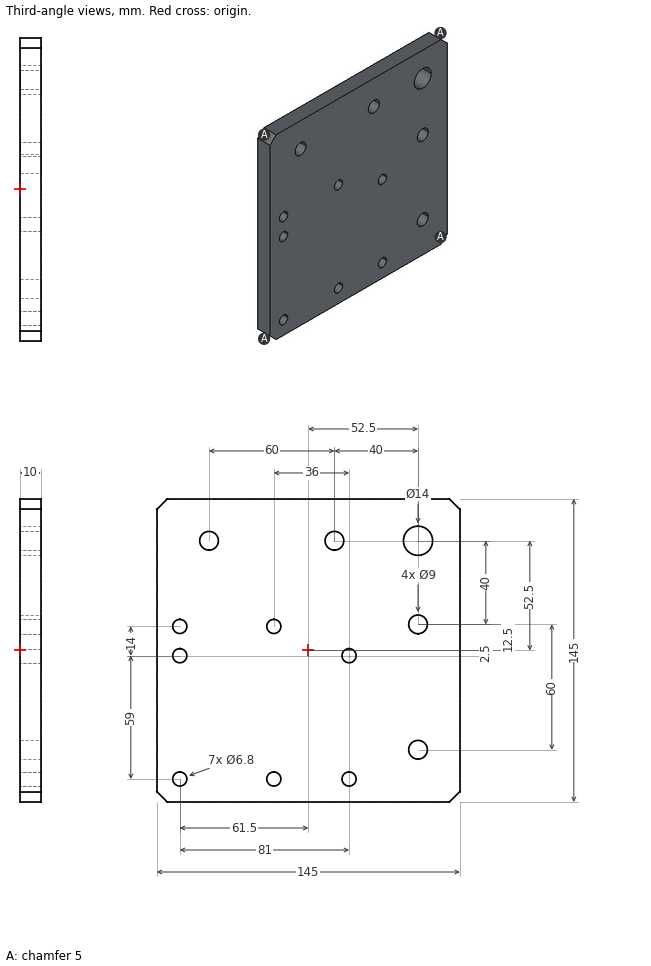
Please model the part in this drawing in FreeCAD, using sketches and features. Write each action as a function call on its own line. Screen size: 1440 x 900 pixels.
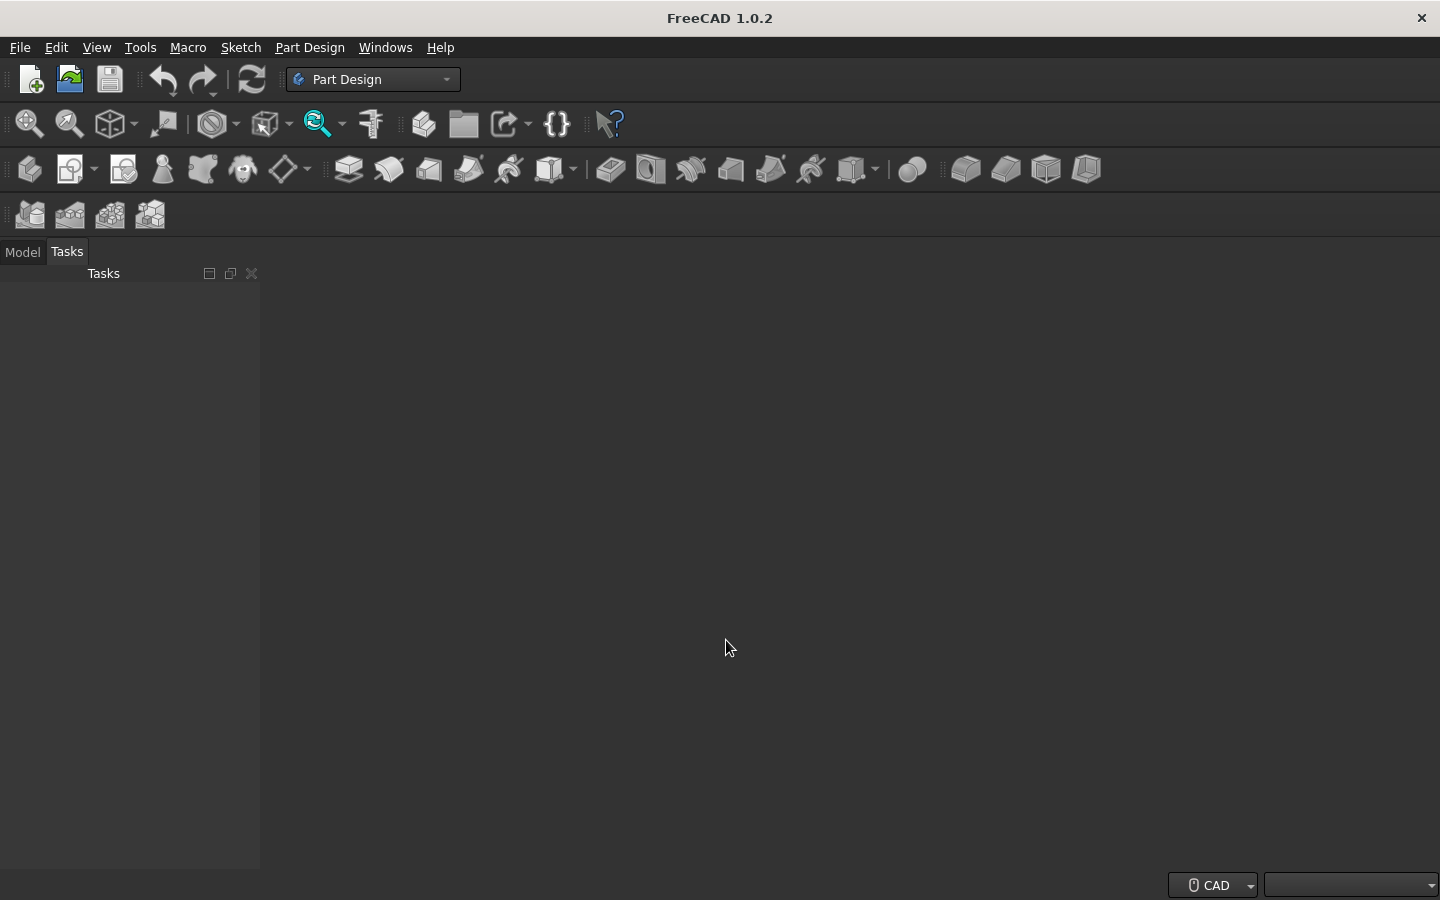
click(30, 80)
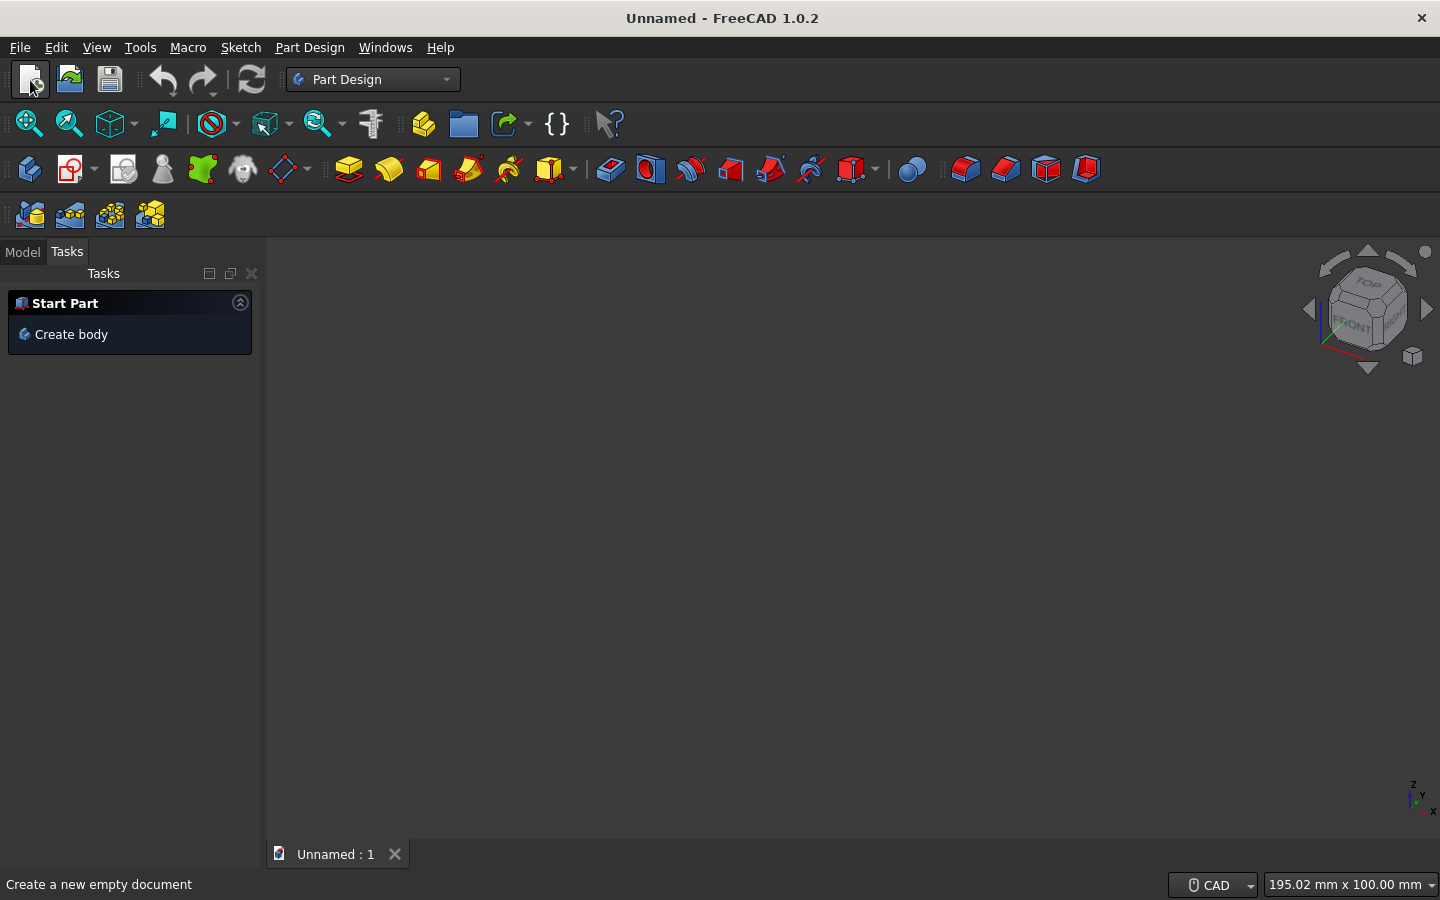
click(70, 170)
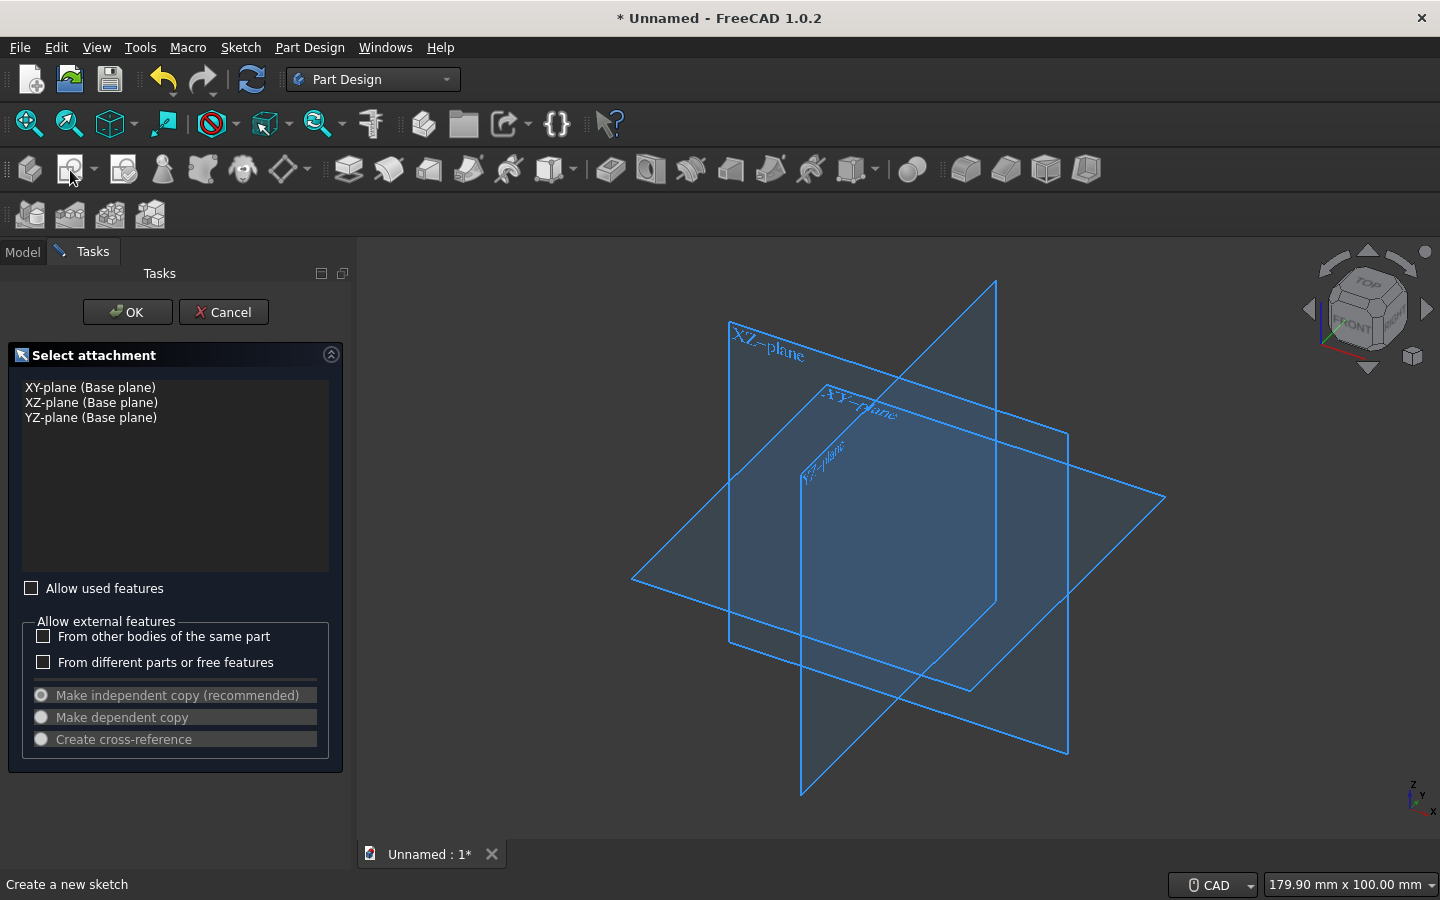
click(82, 418)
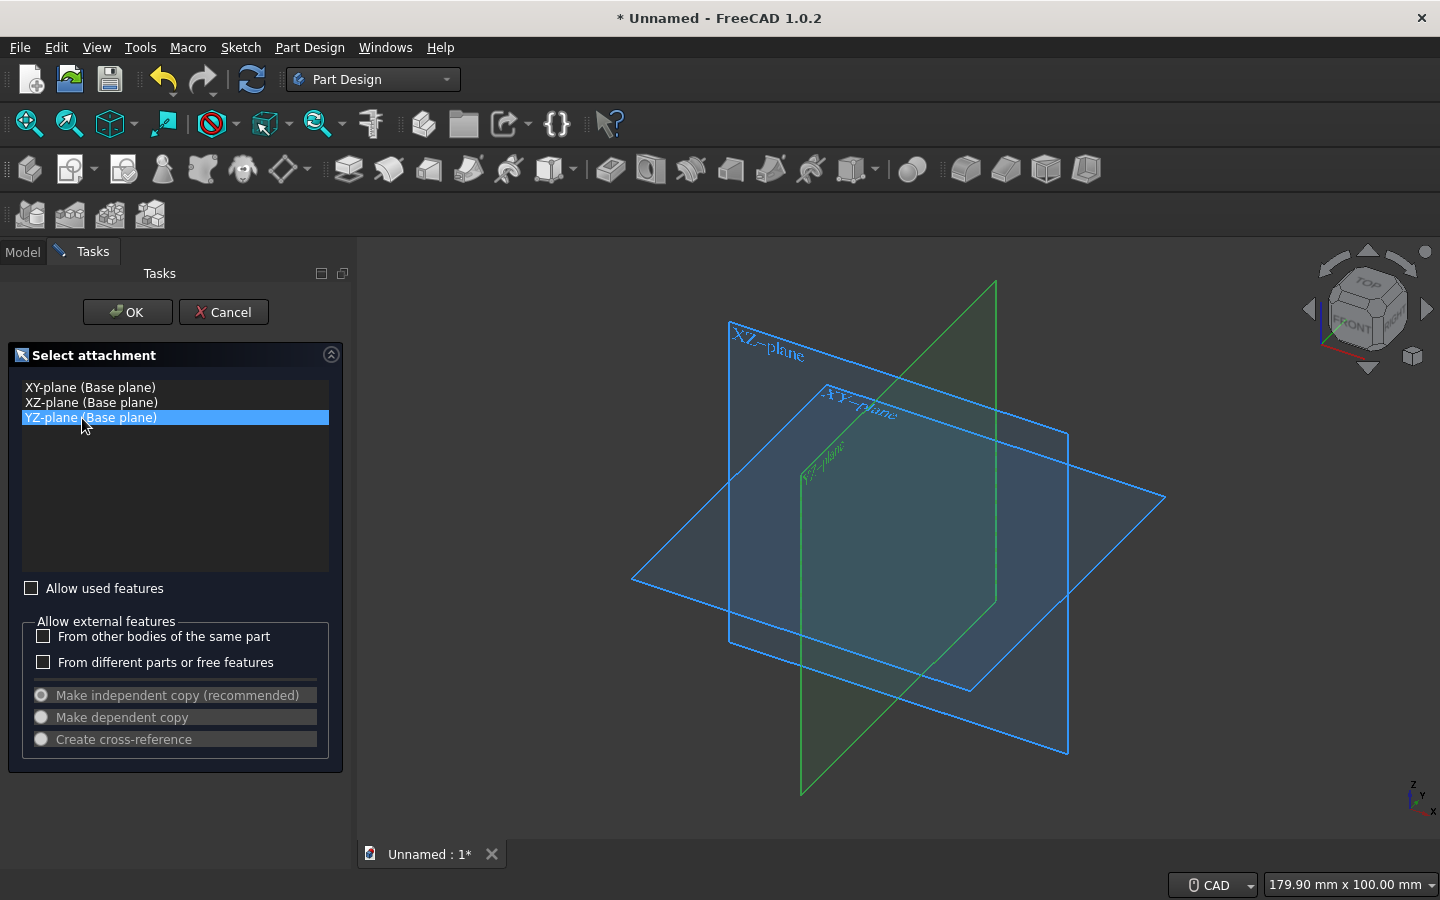
click(128, 312)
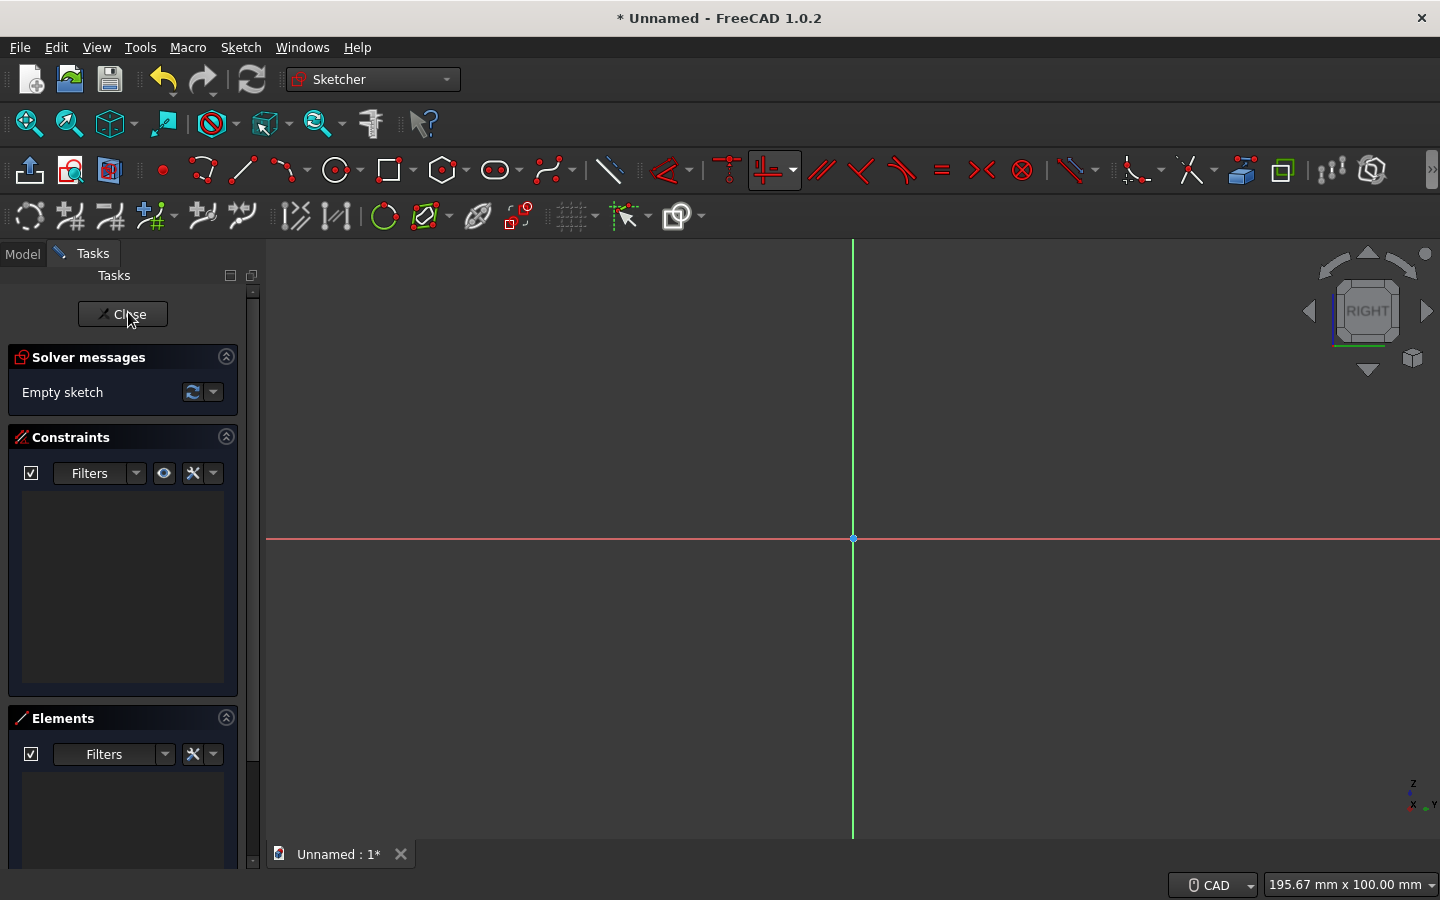
scroll(729, 539, down, 4)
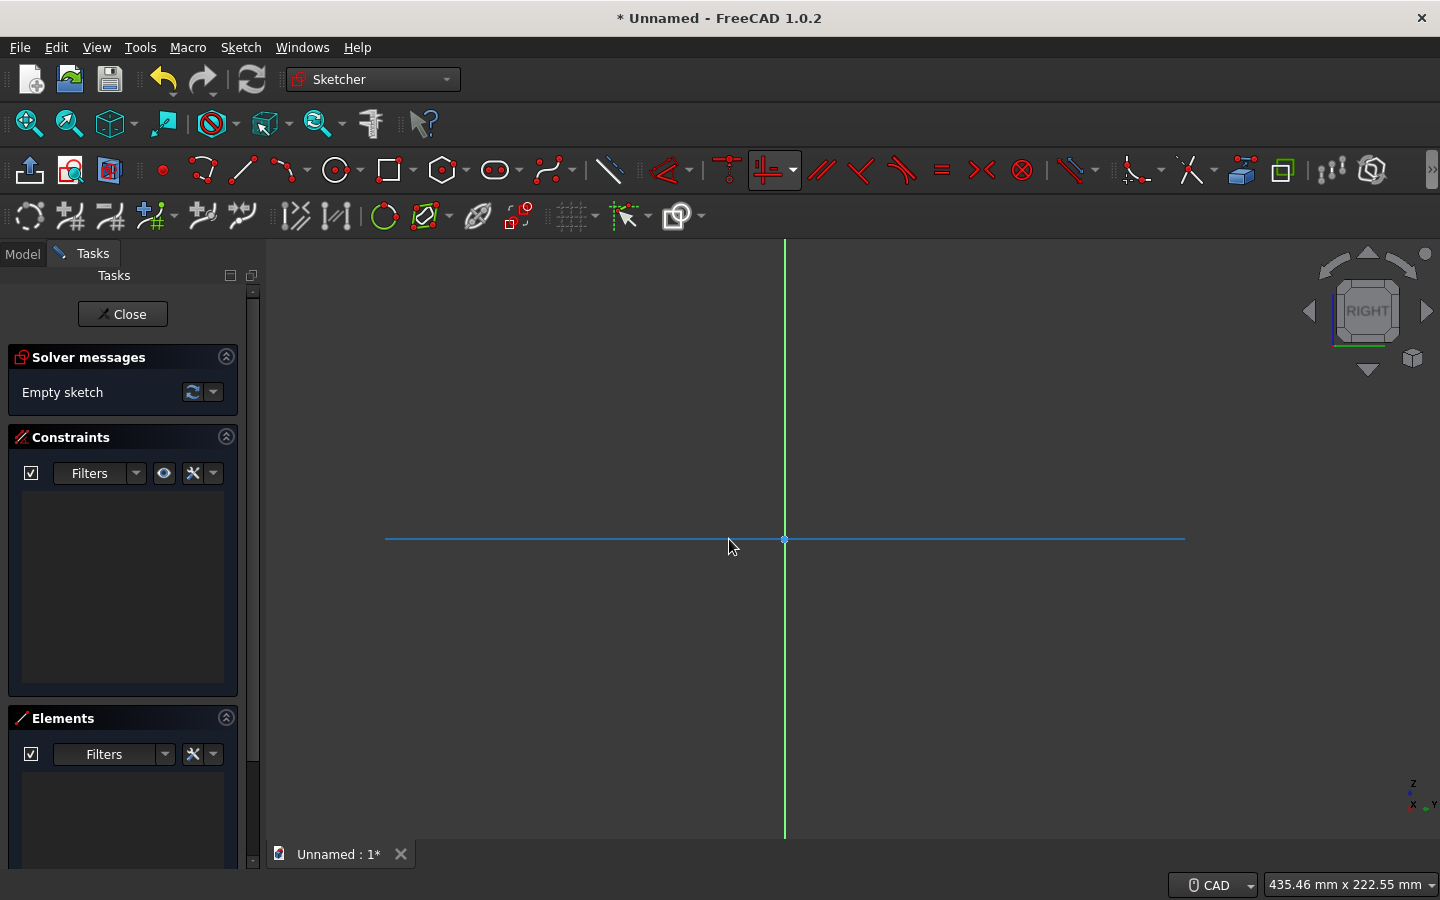
click(416, 170)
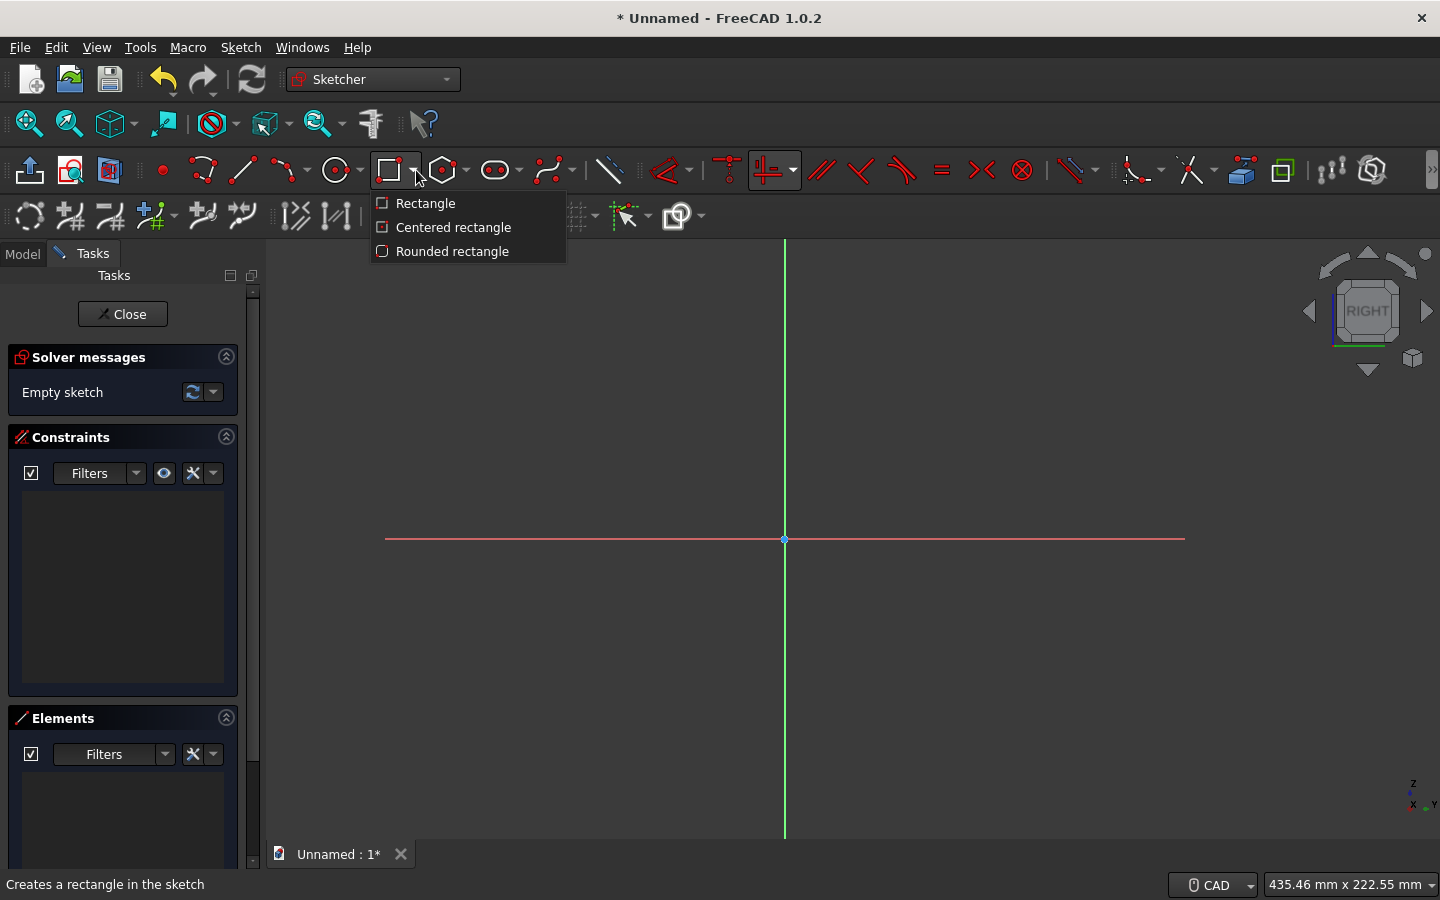
click(468, 227)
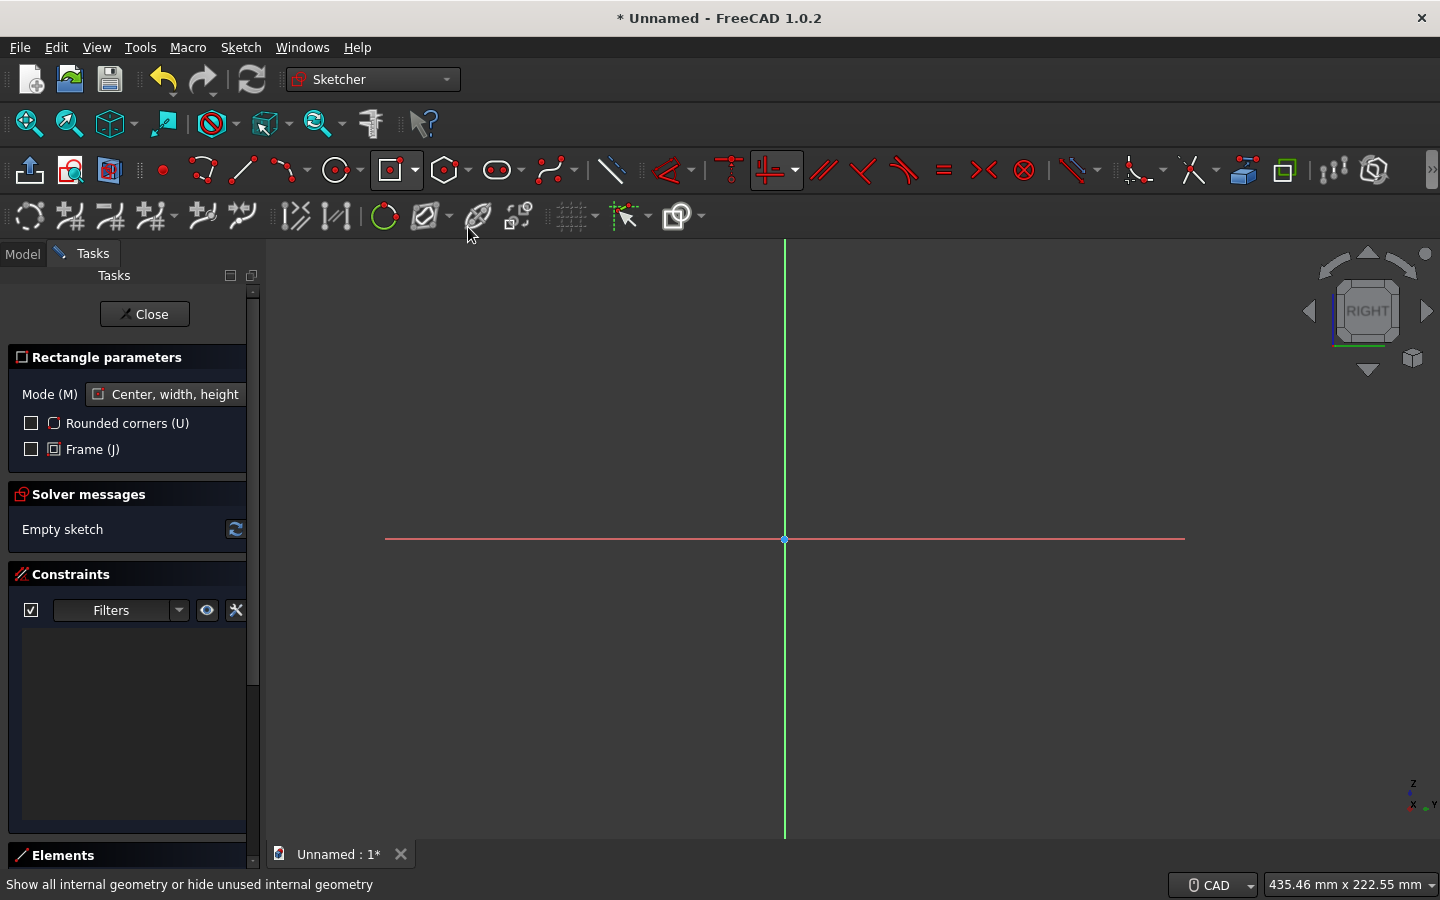
click(785, 539)
click(980, 344)
key(Escape)